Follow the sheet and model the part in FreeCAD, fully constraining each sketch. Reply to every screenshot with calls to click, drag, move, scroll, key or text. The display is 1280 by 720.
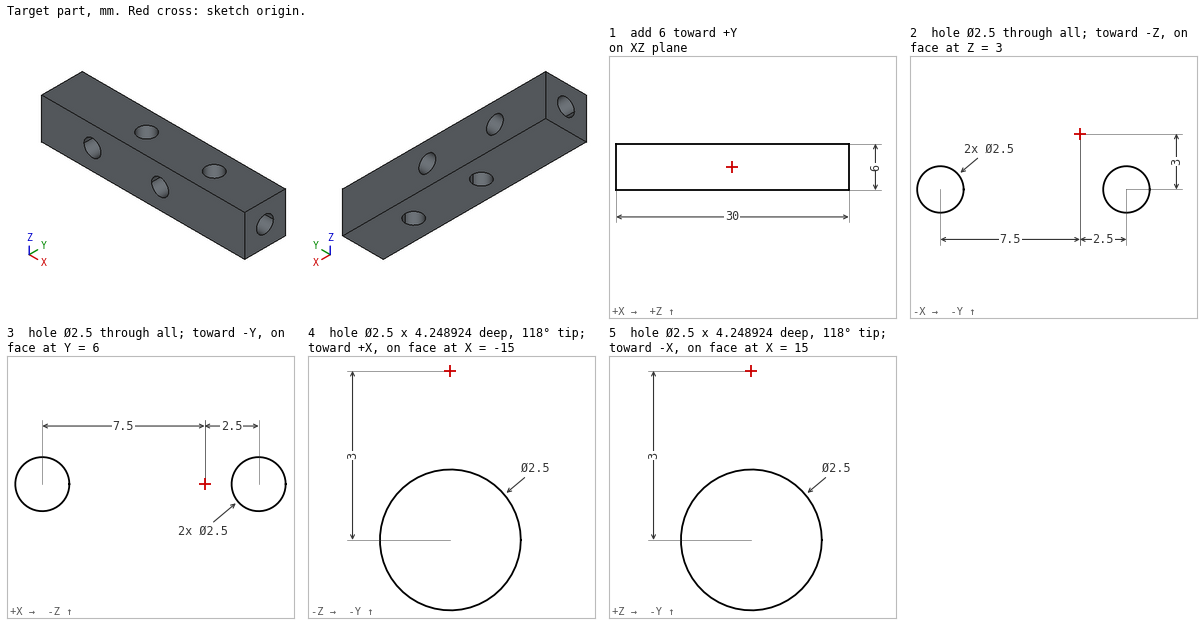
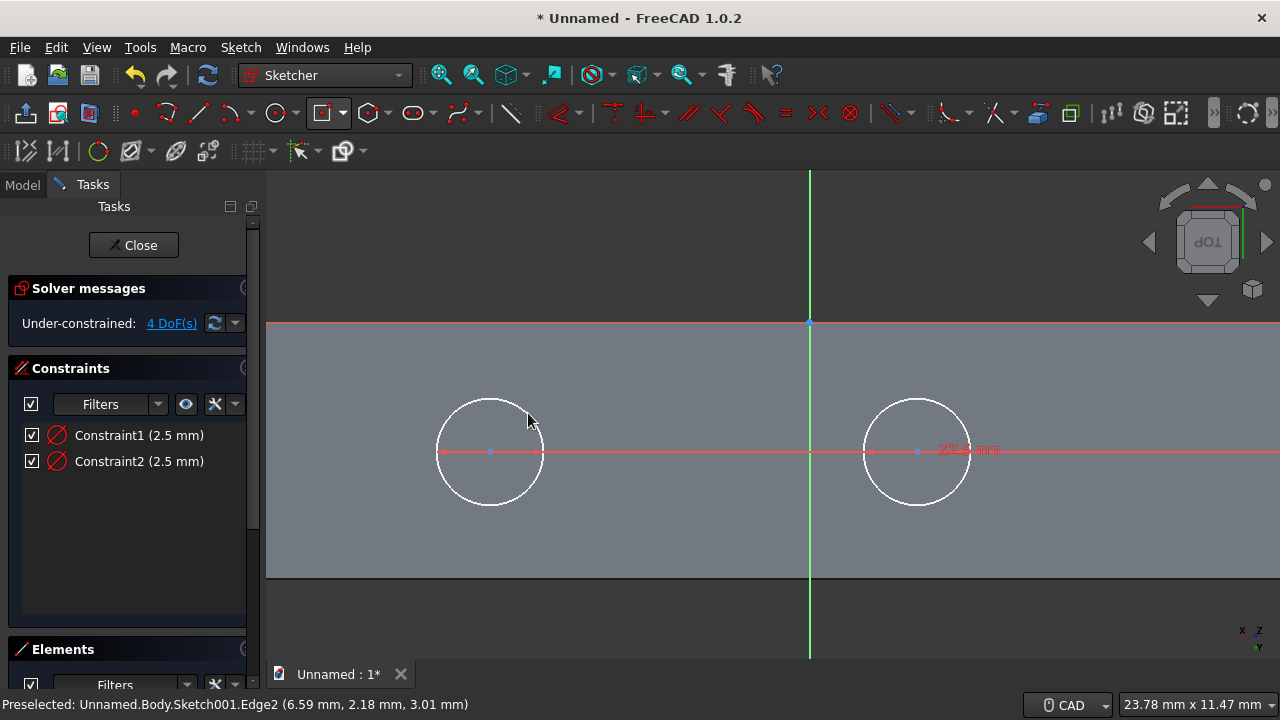
click(917, 452)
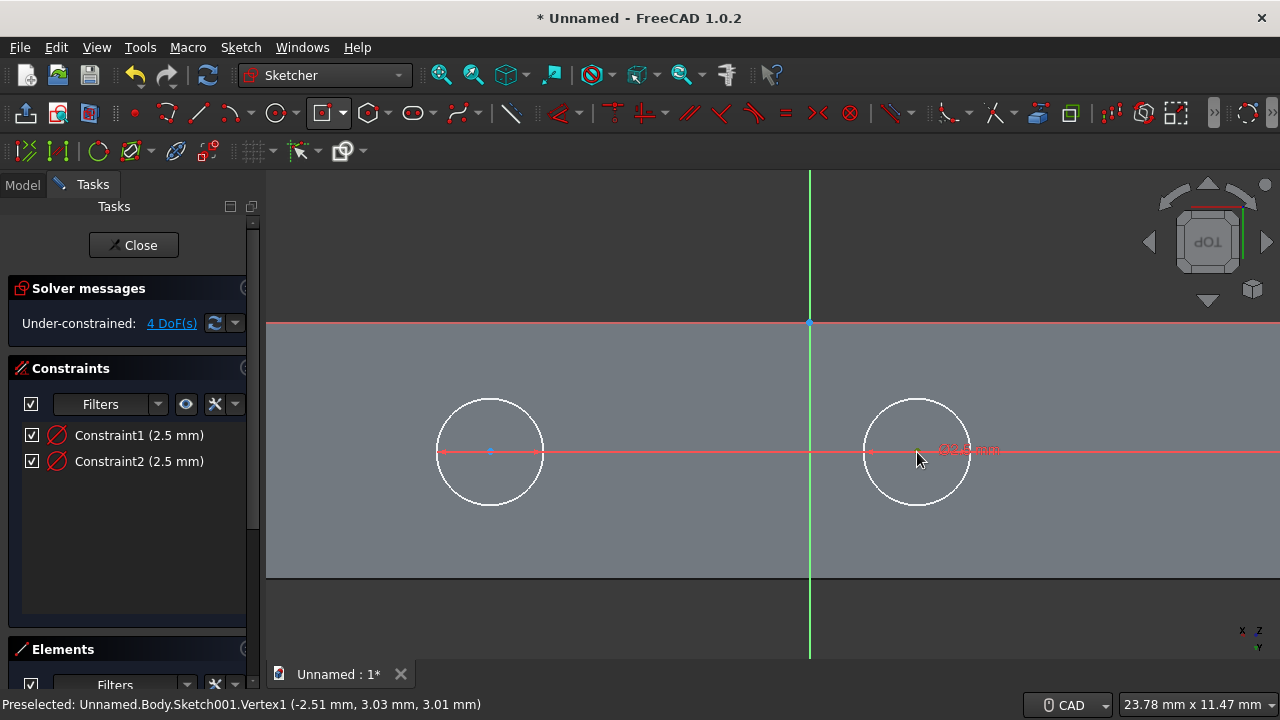
click(490, 452)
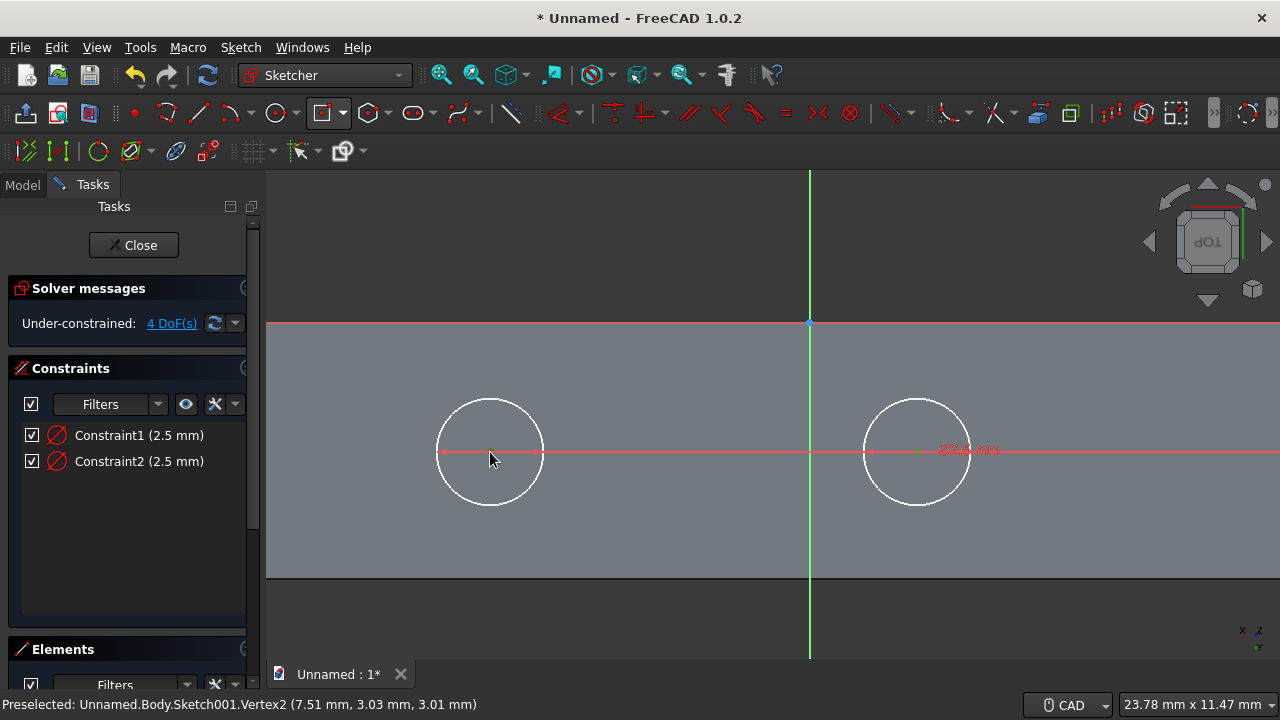
key(h)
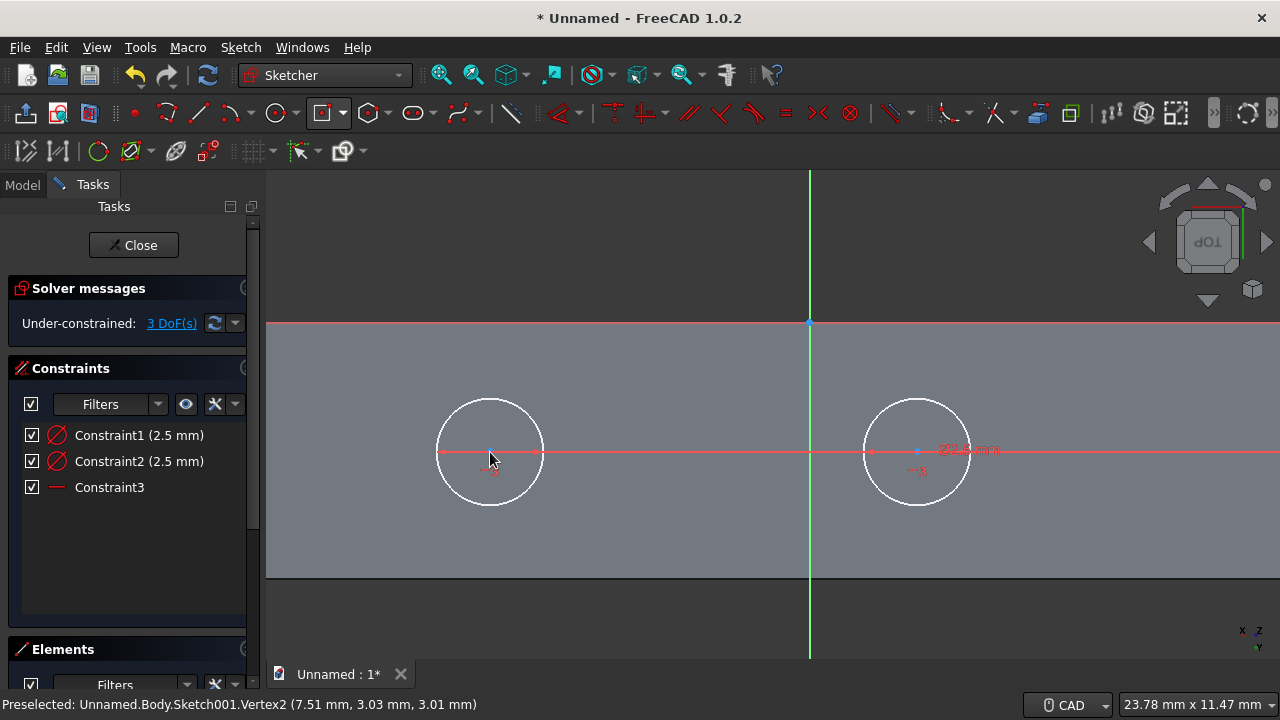
click(917, 452)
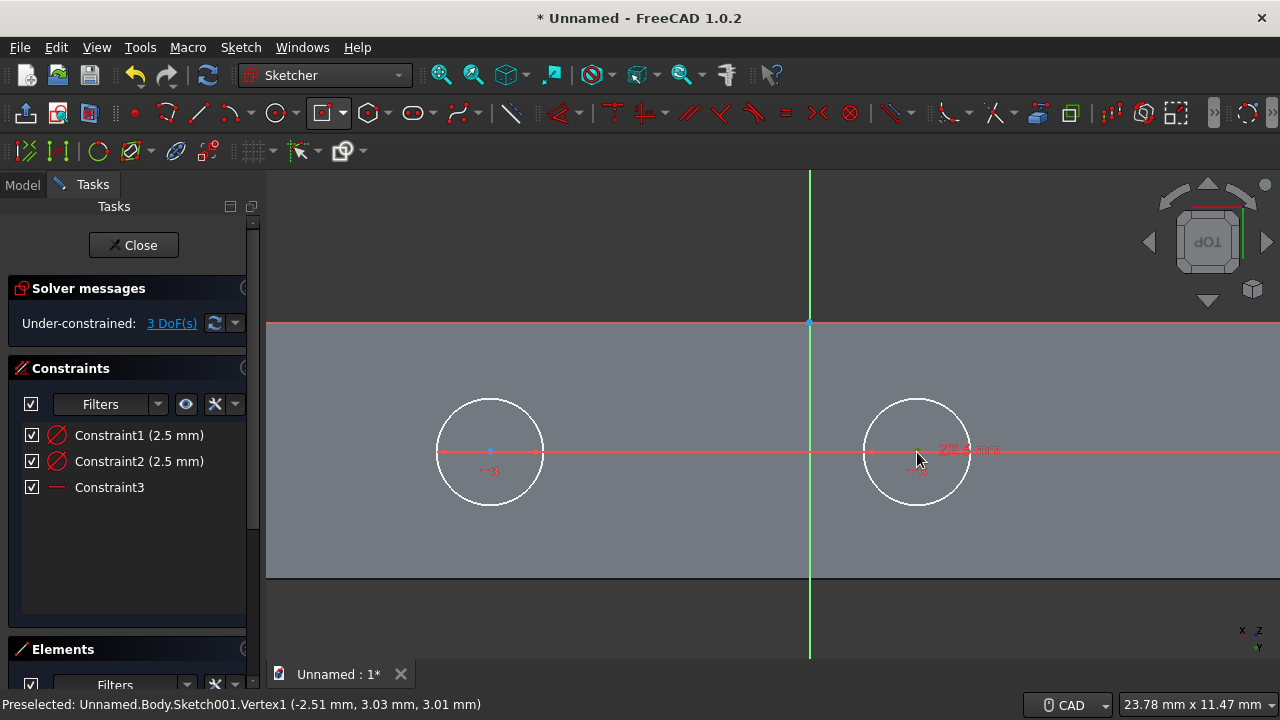
click(582, 114)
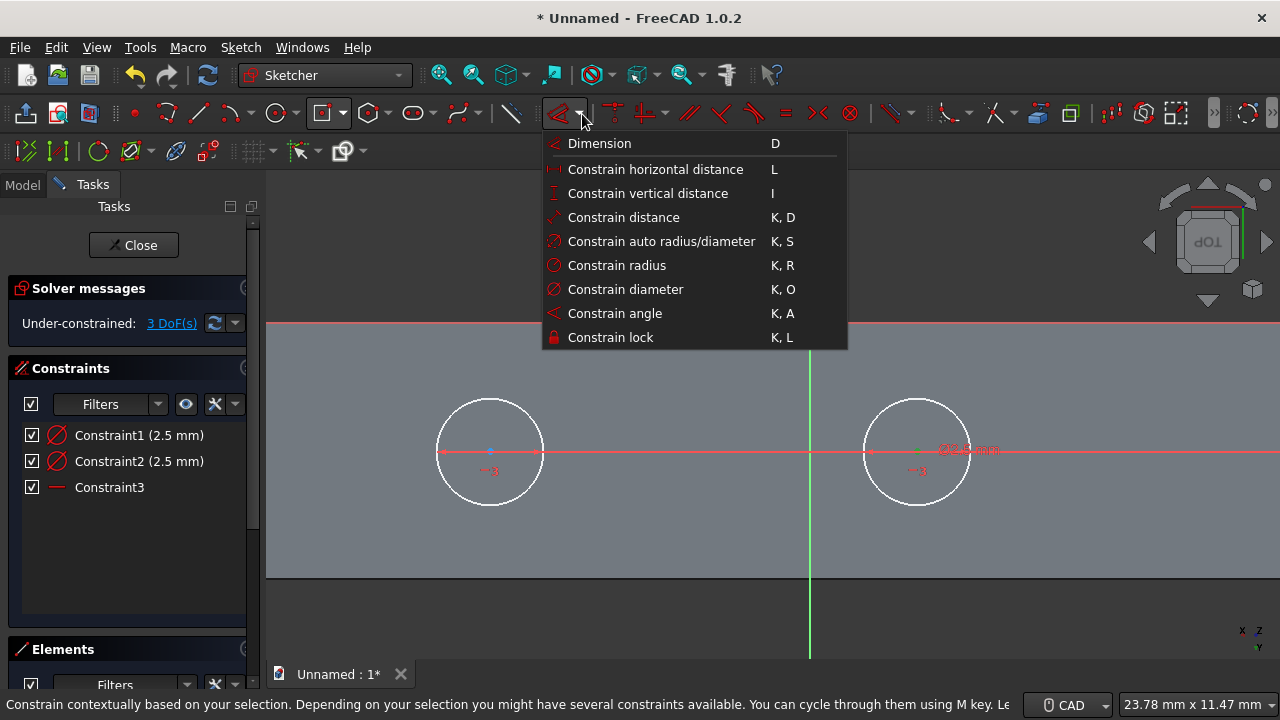
click(695, 193)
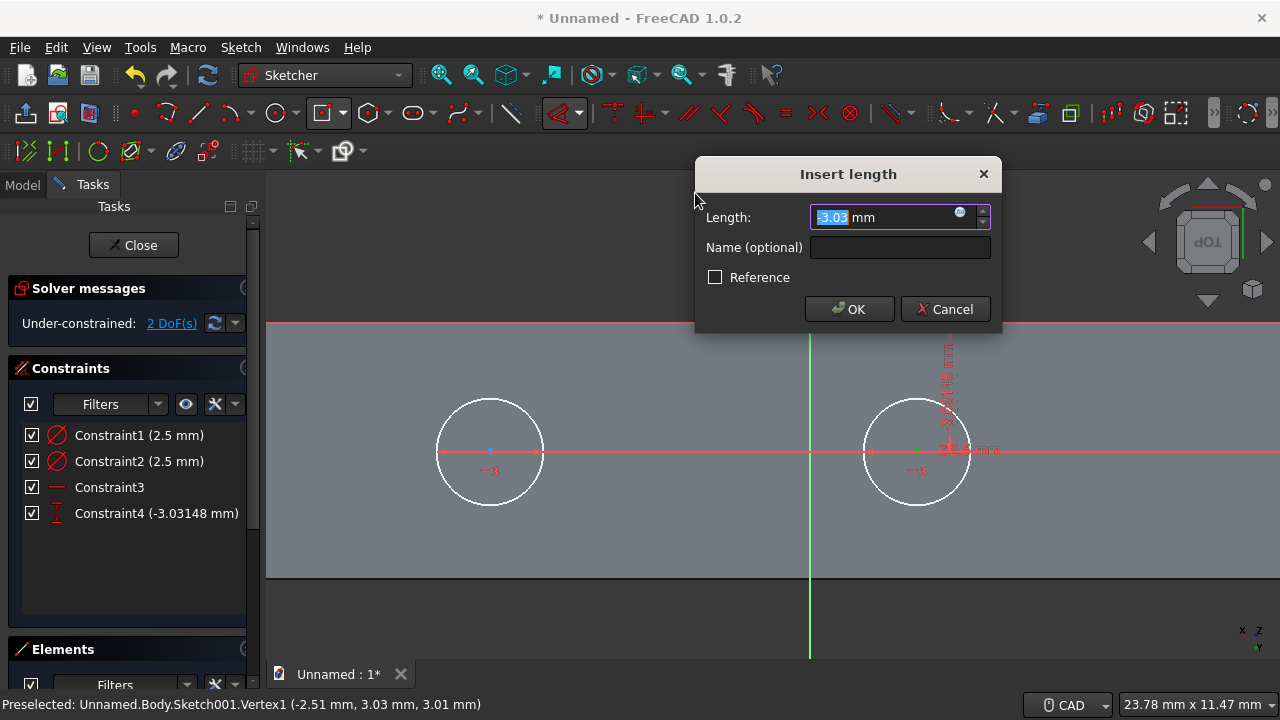
text(-3)
key(Return)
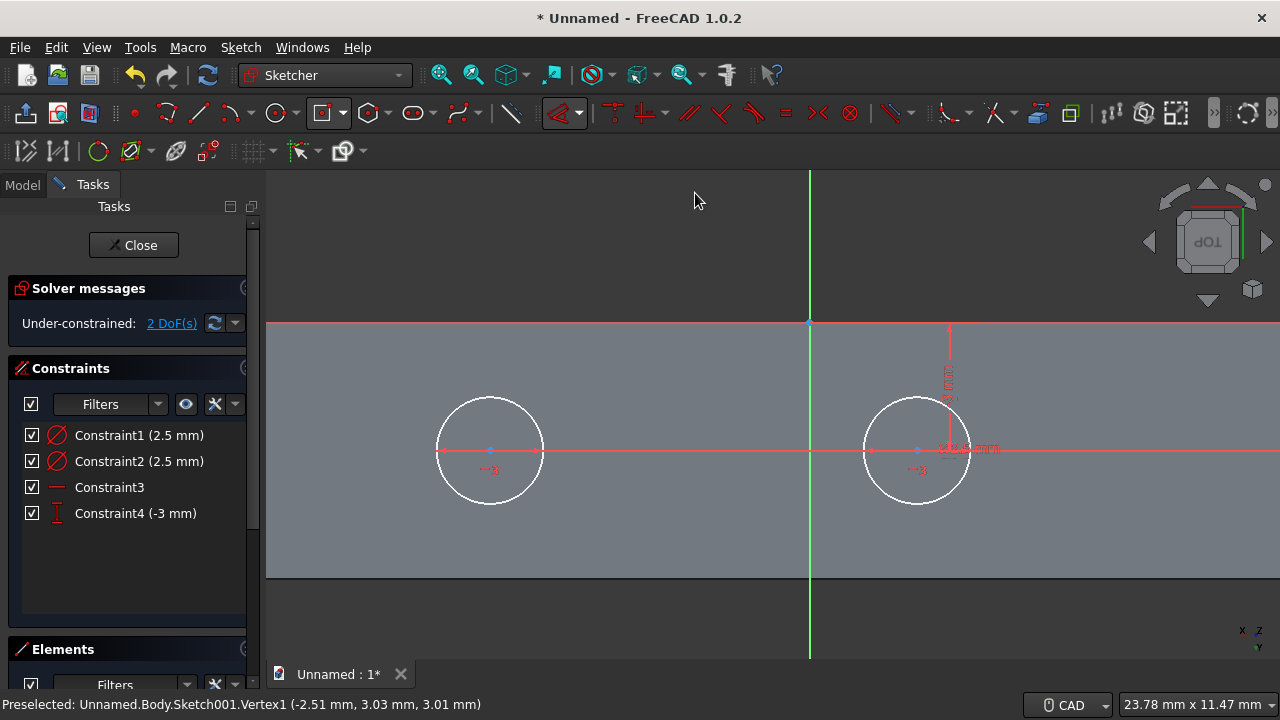
click(917, 451)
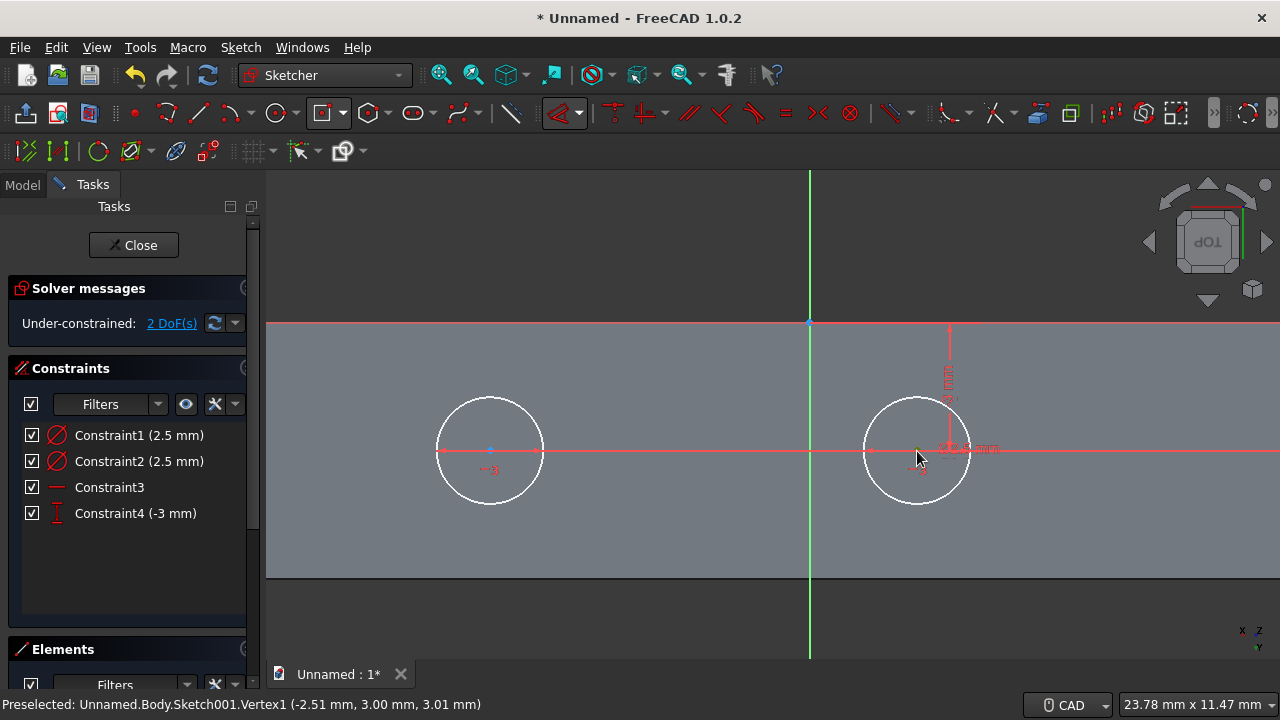
key(l)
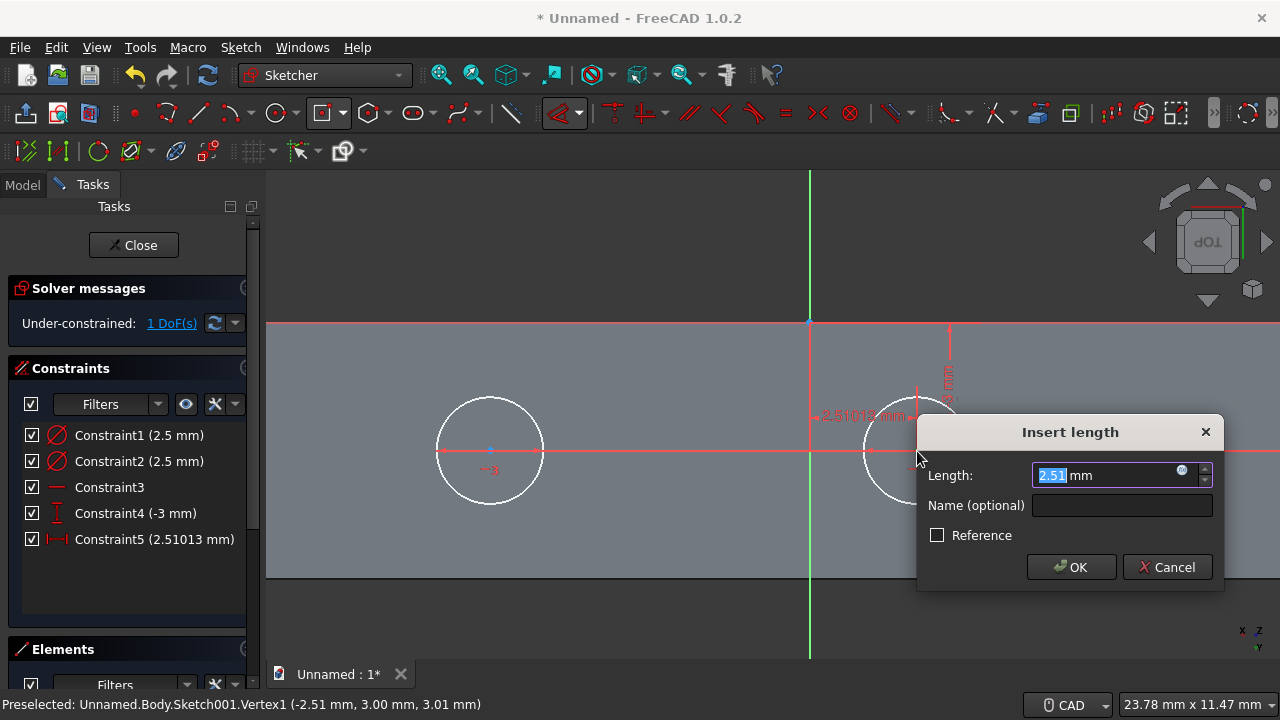
text(2.5)
key(Return)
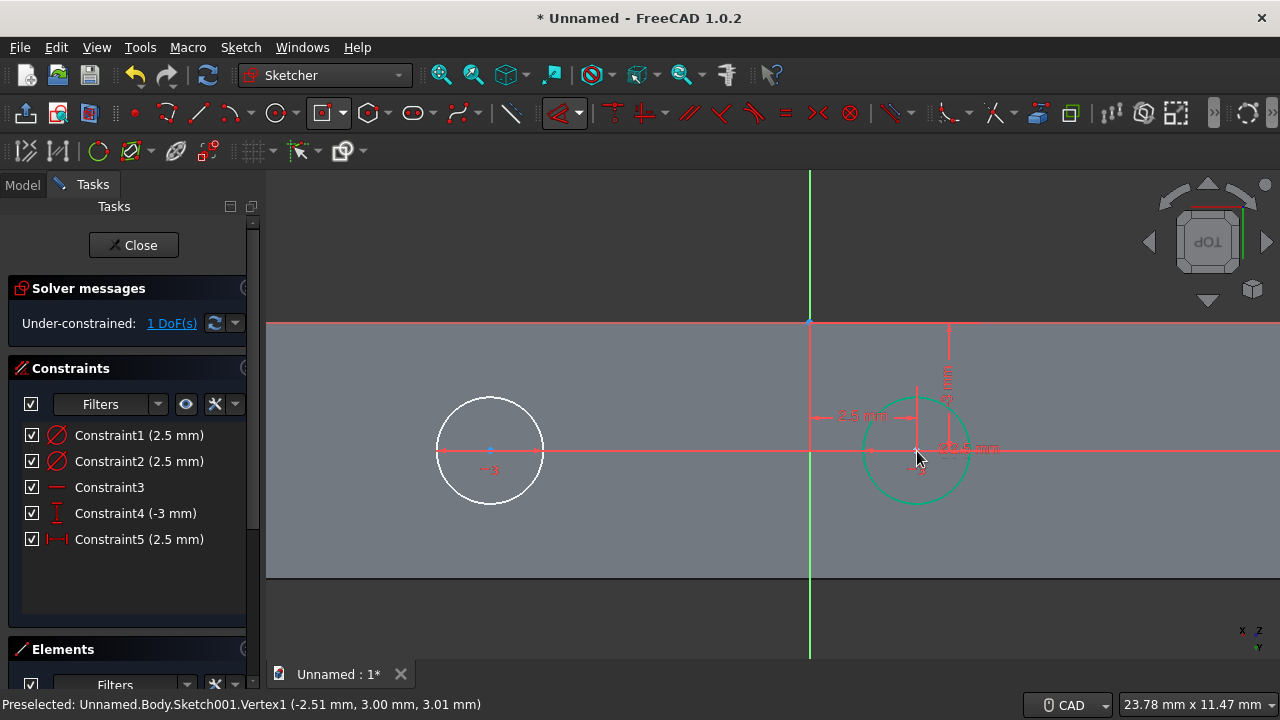
click(490, 451)